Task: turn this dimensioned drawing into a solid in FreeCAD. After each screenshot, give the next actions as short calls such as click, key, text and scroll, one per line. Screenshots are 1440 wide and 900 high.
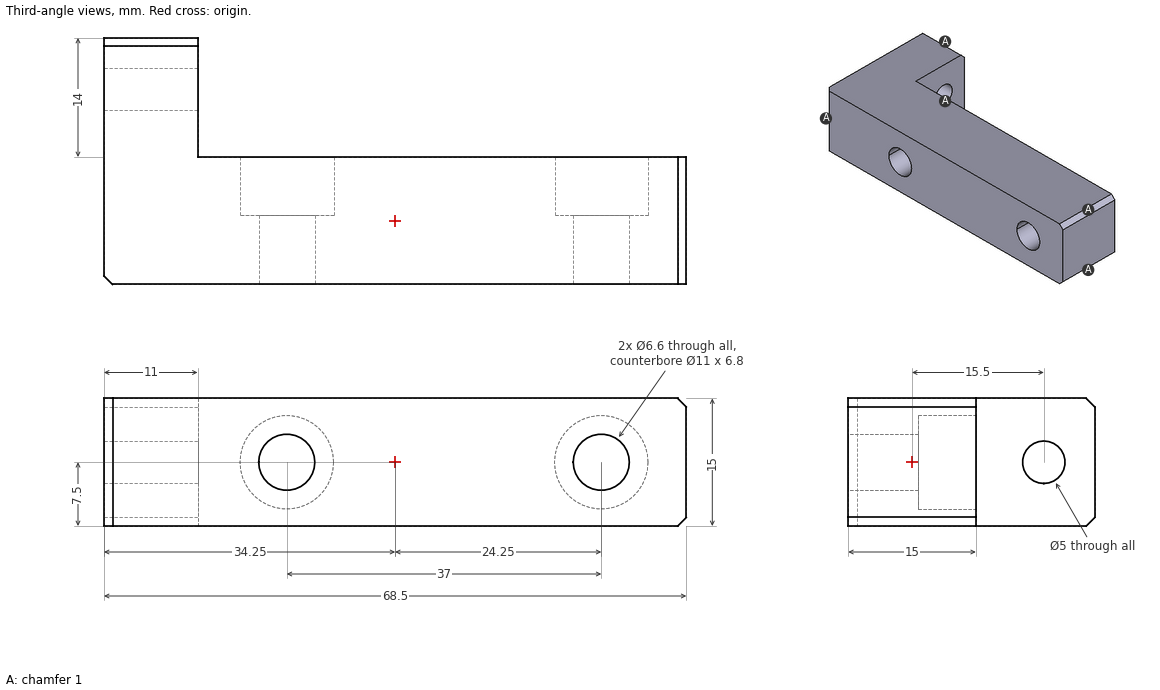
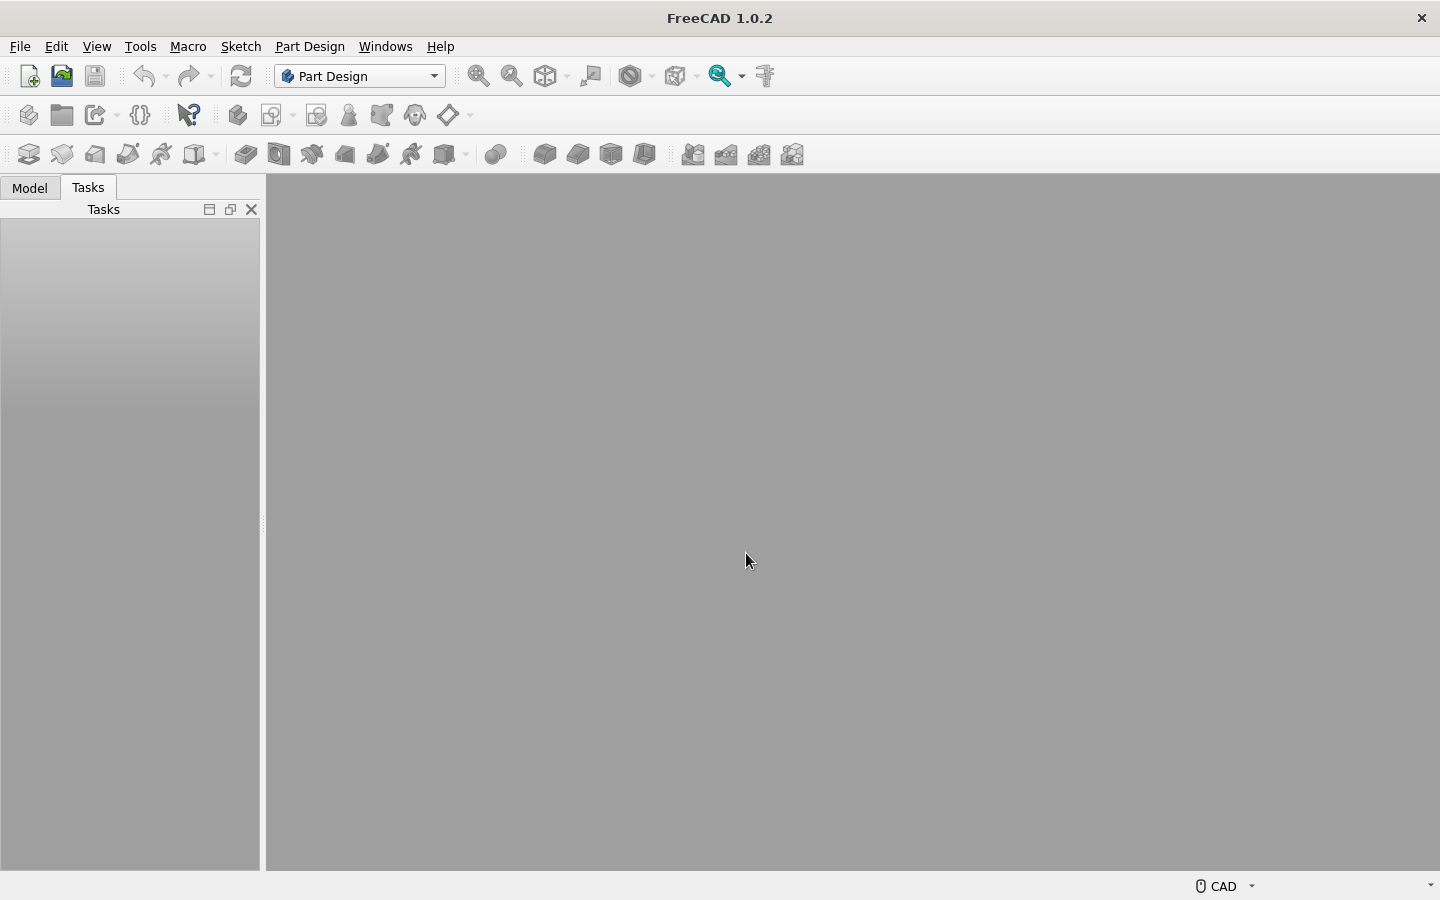
click(29, 76)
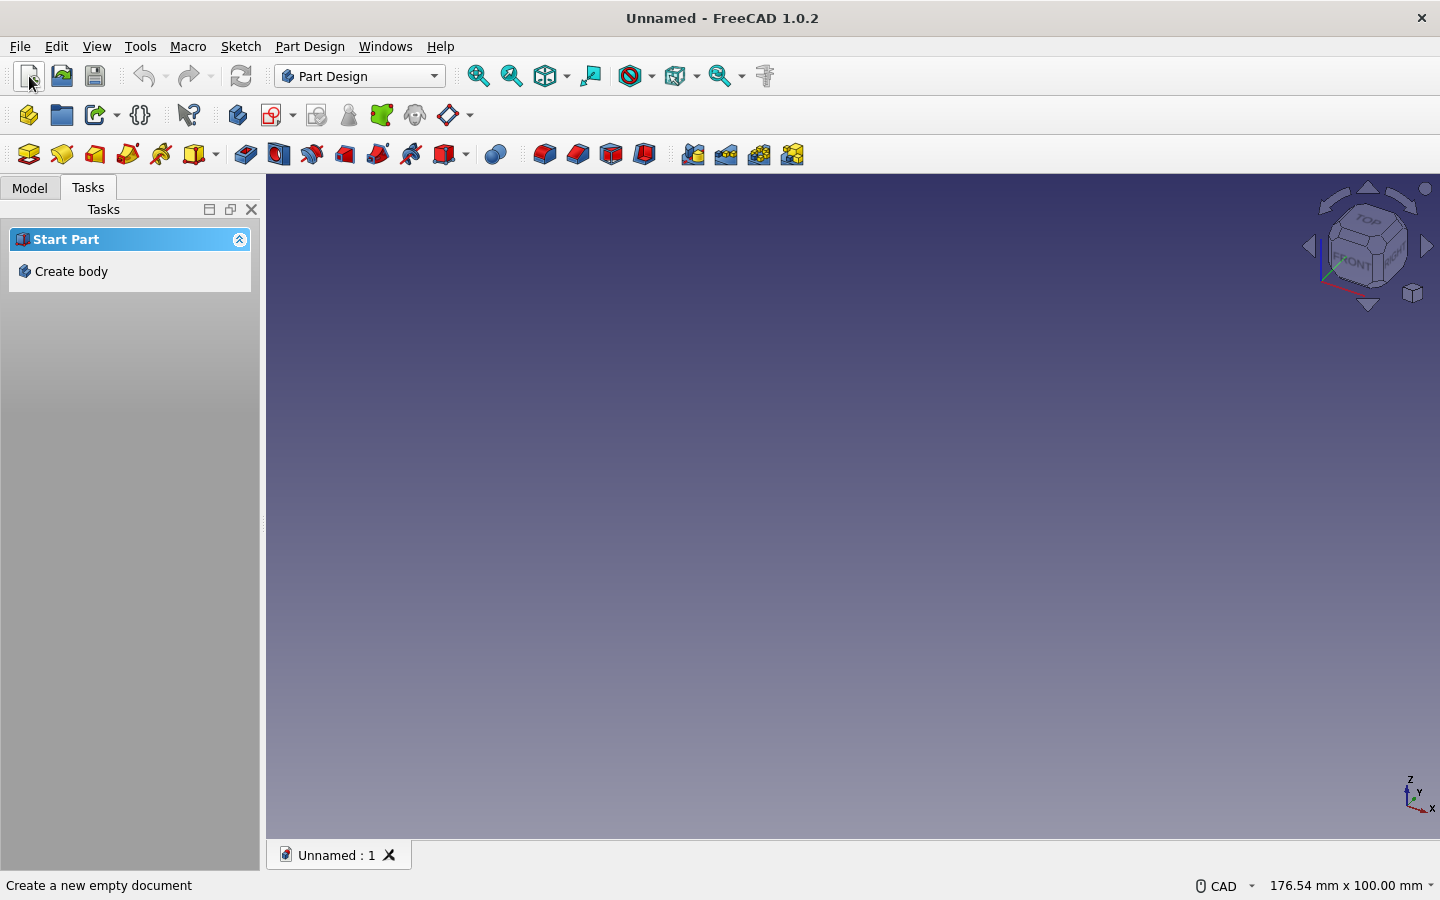
click(270, 116)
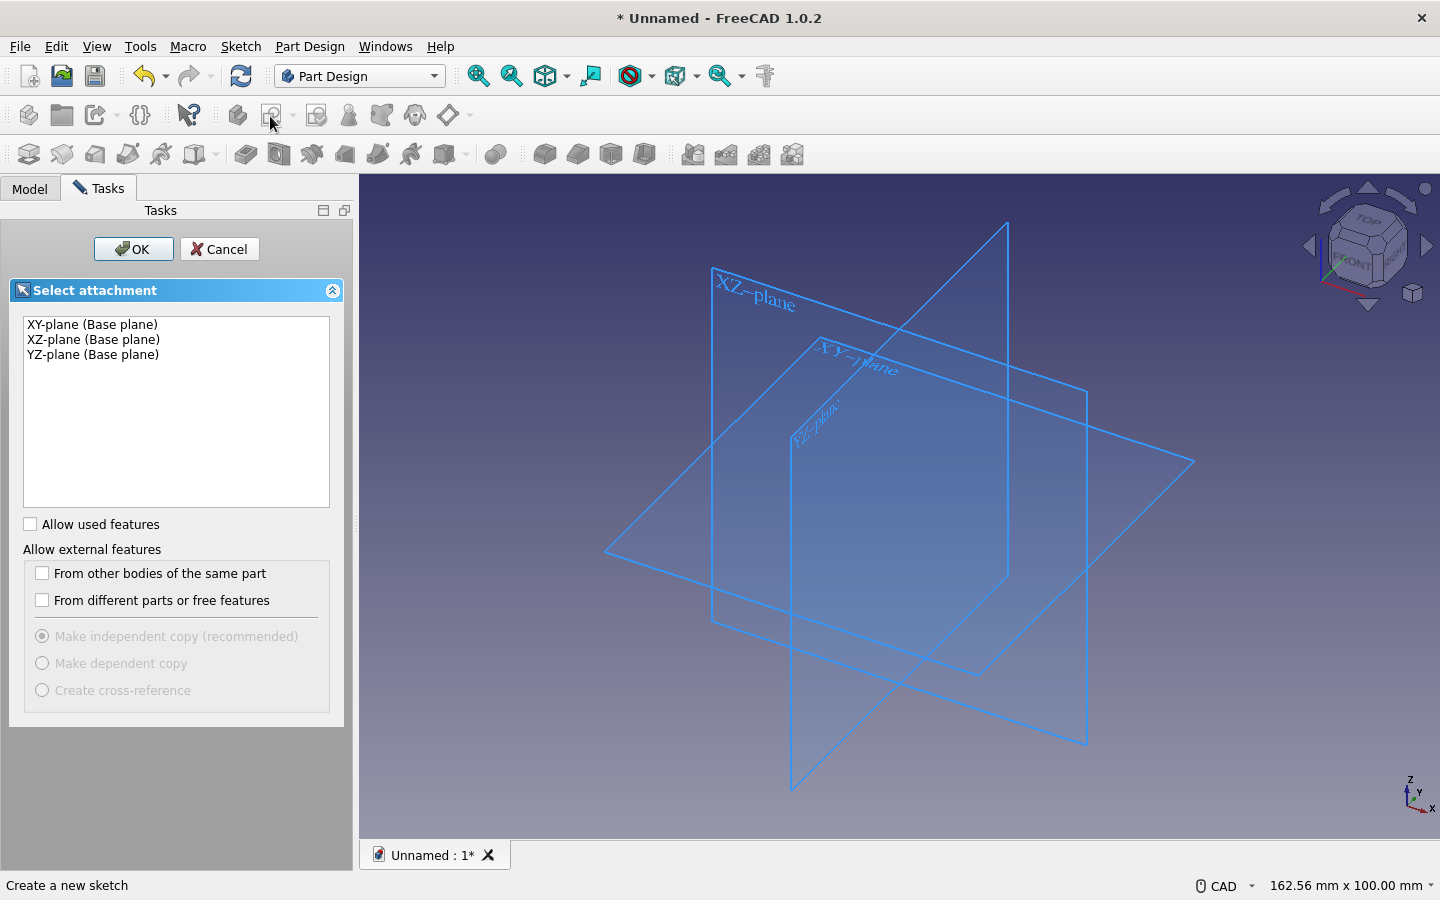
click(84, 340)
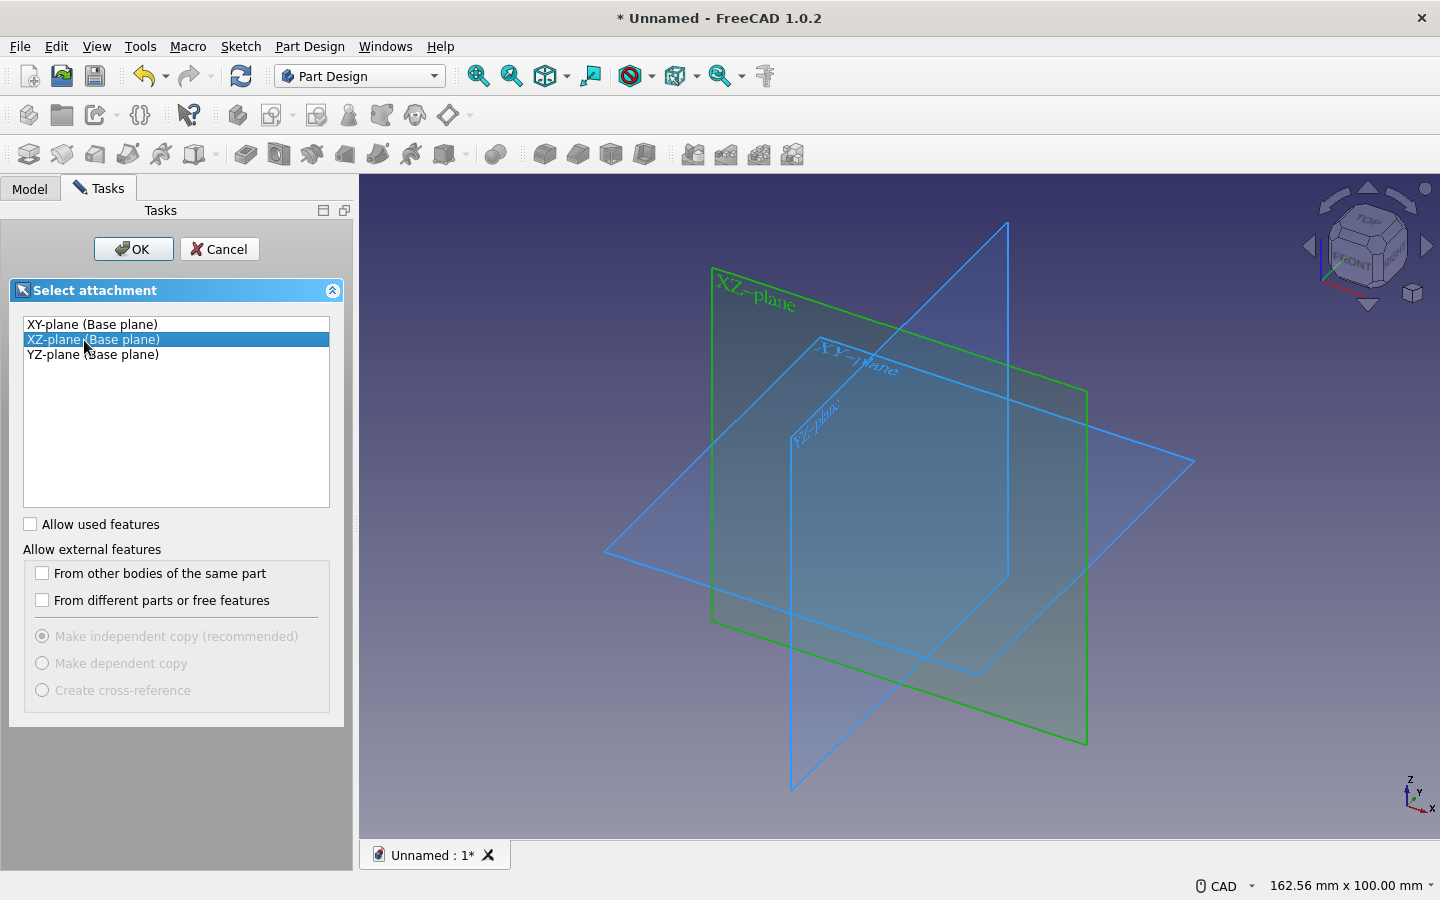
click(134, 249)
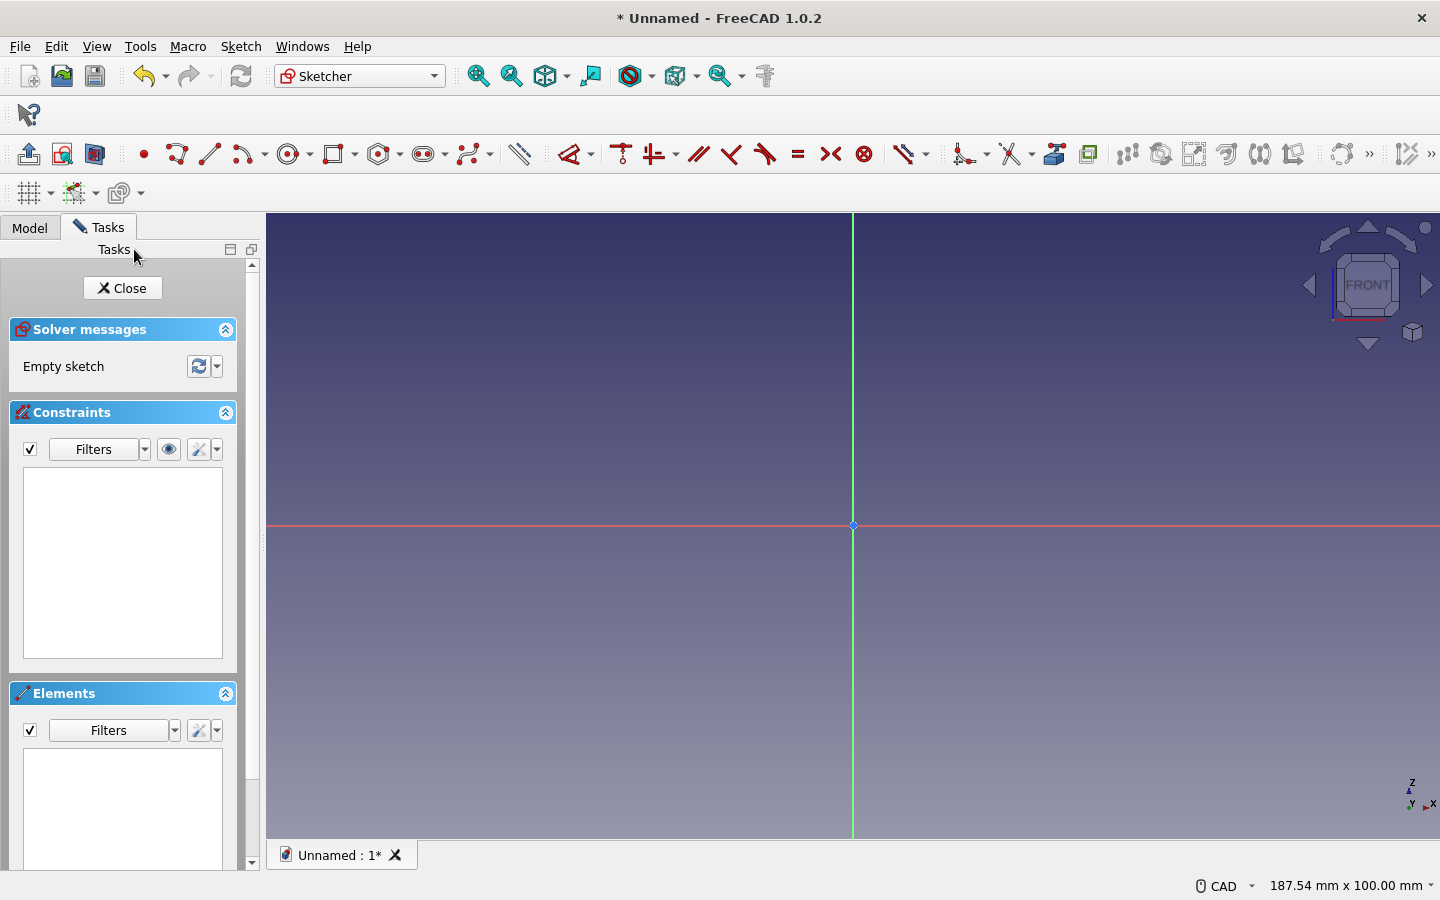
scroll(992, 526, up, 2)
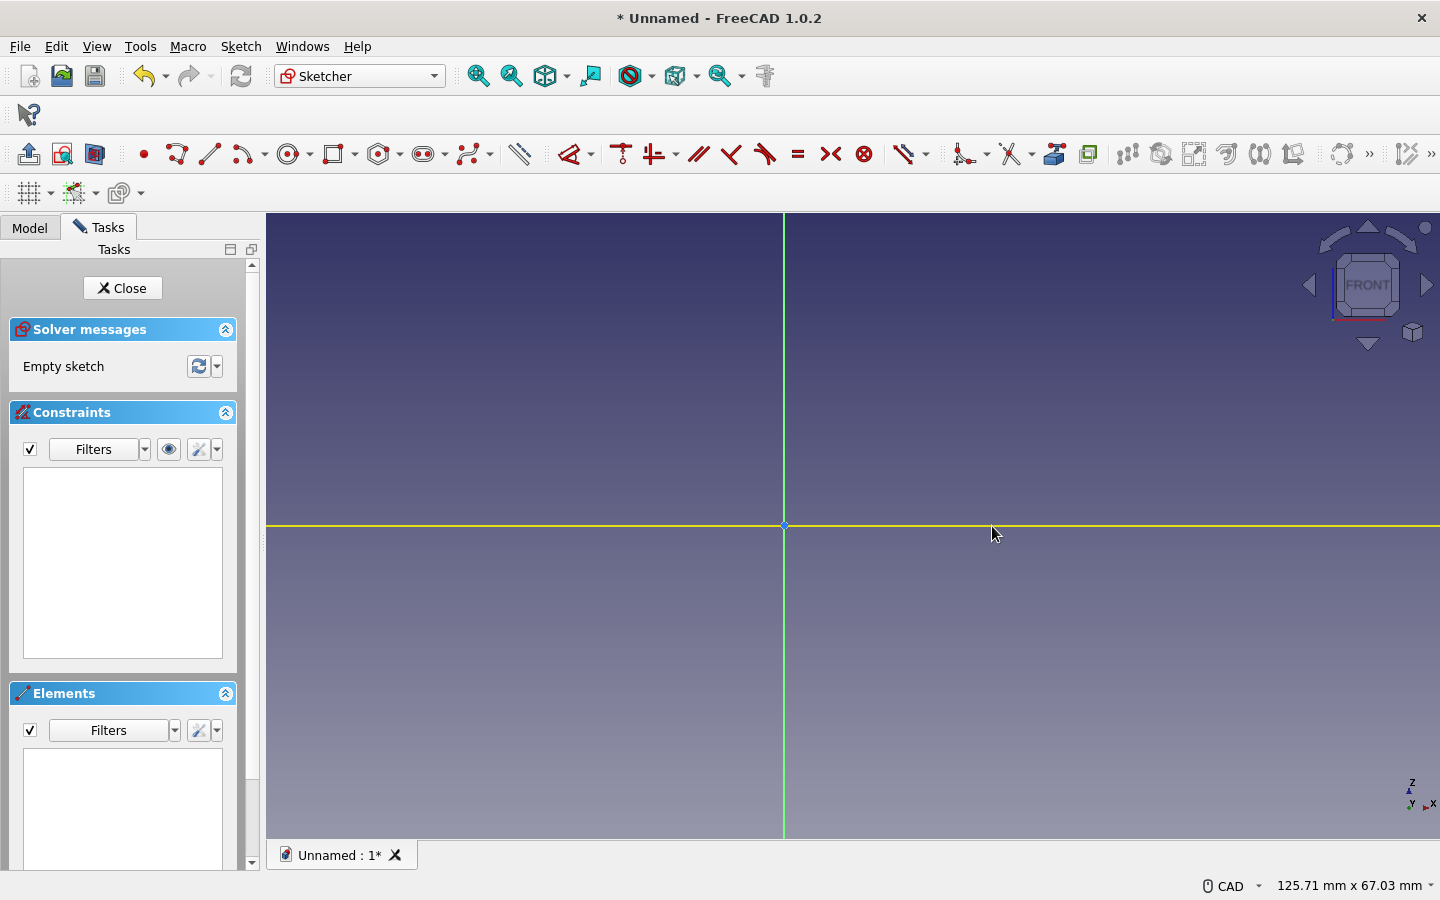
key(g)
key(v)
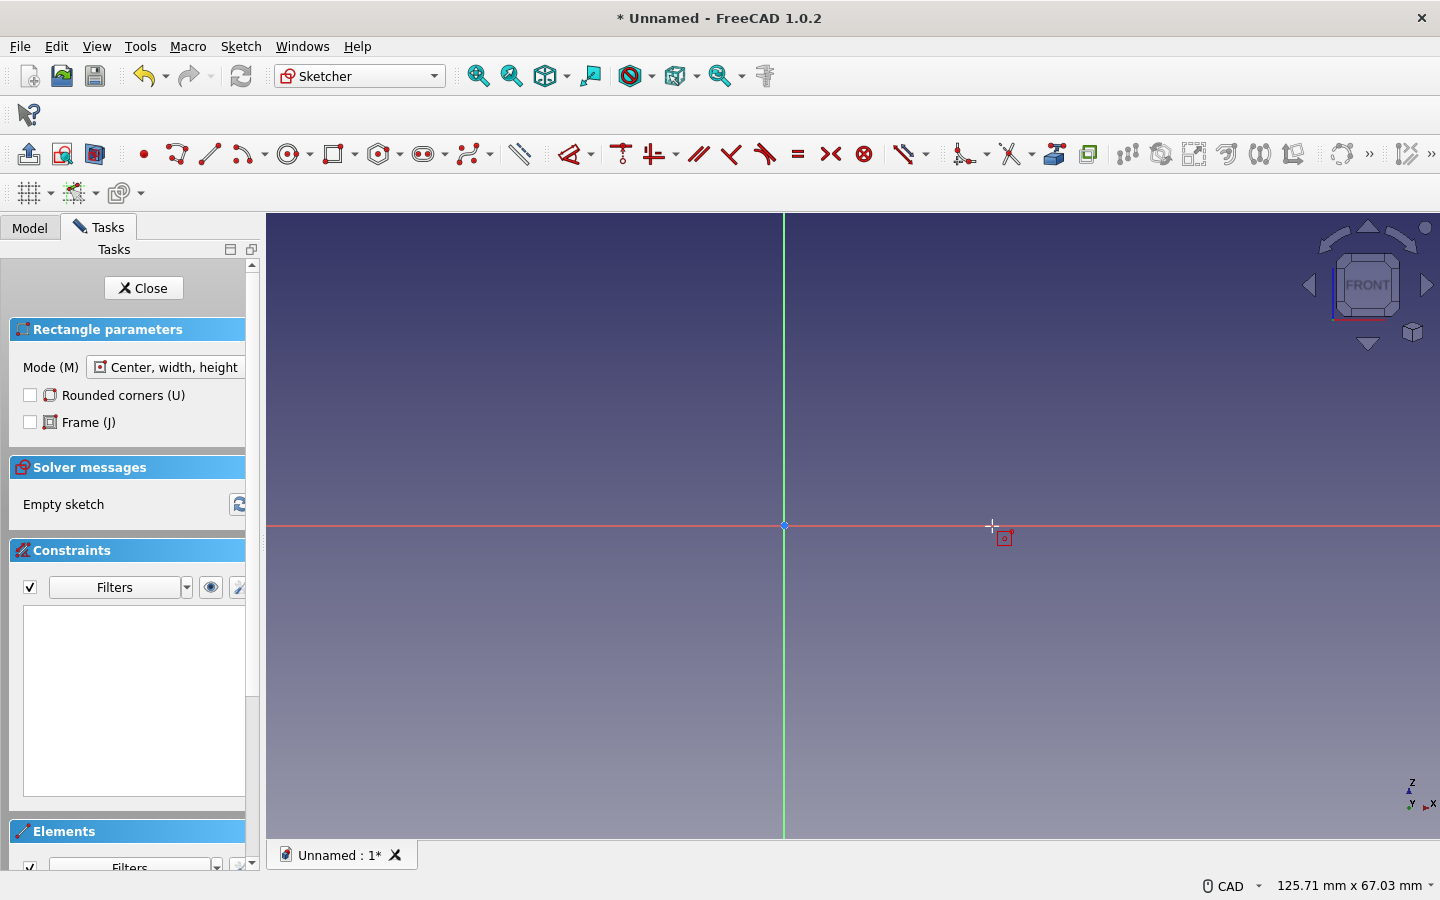
click(784, 526)
move(1104, 456)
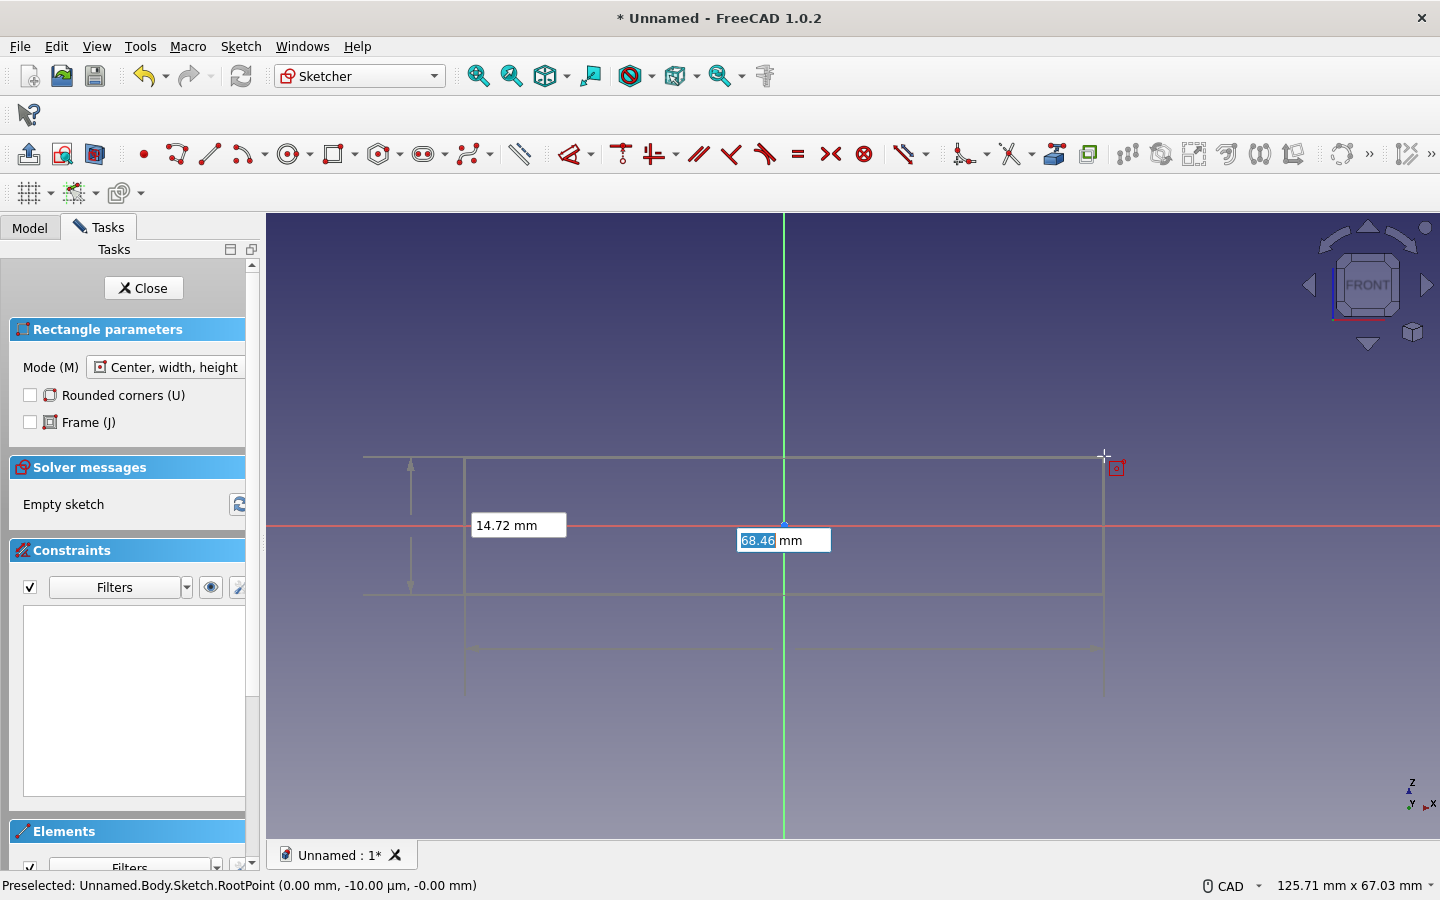
text(68.5)
key(Tab)
text(15)
key(Return)
key(Escape)